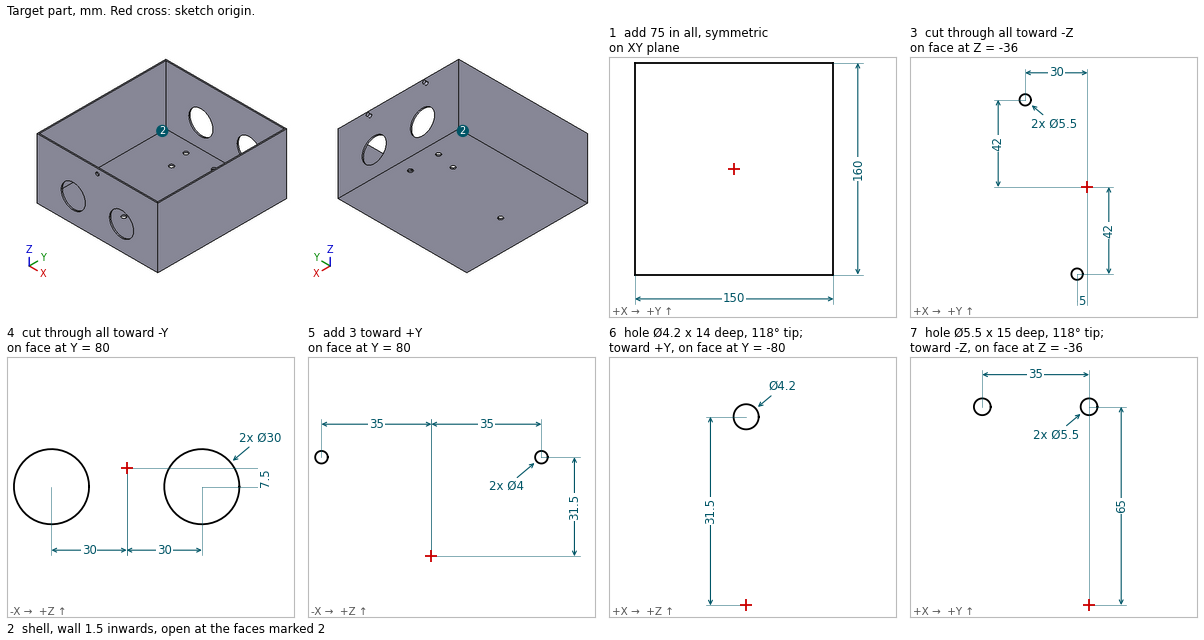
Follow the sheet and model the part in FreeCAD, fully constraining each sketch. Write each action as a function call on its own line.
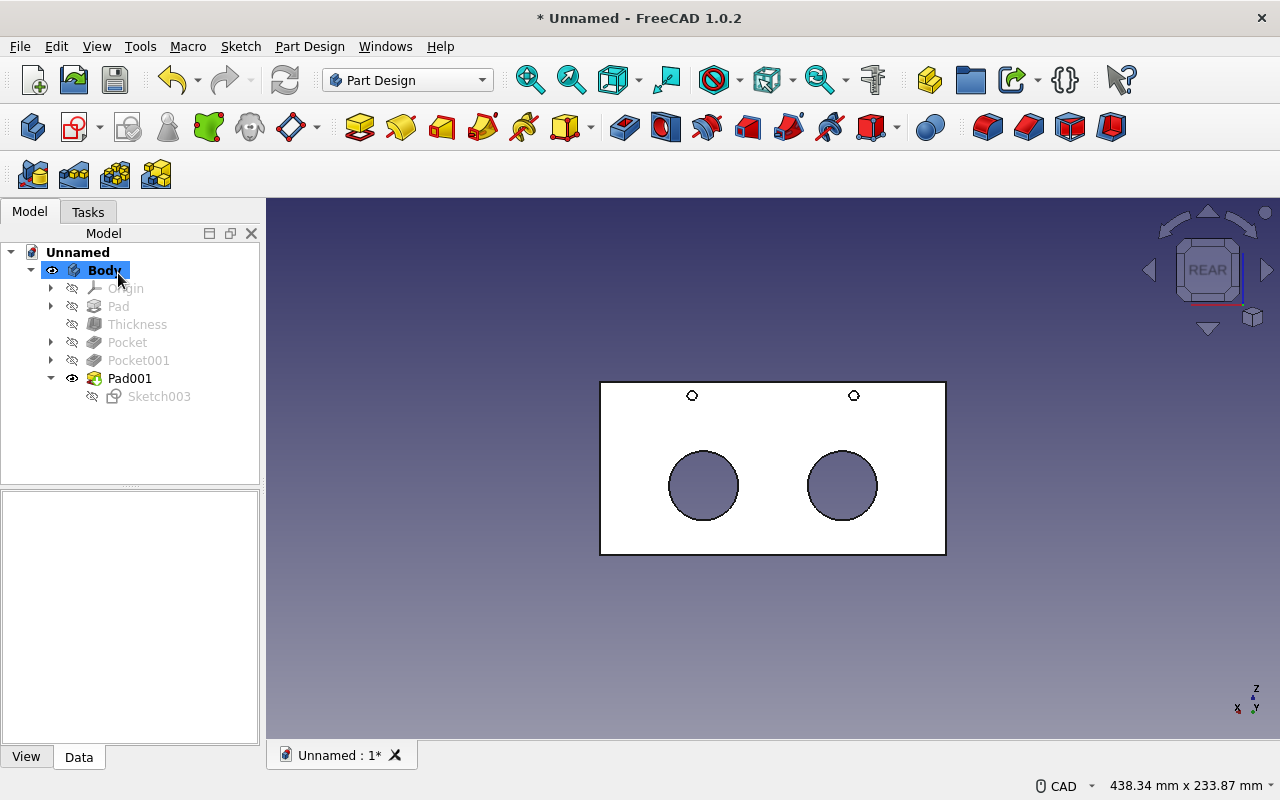
key(0)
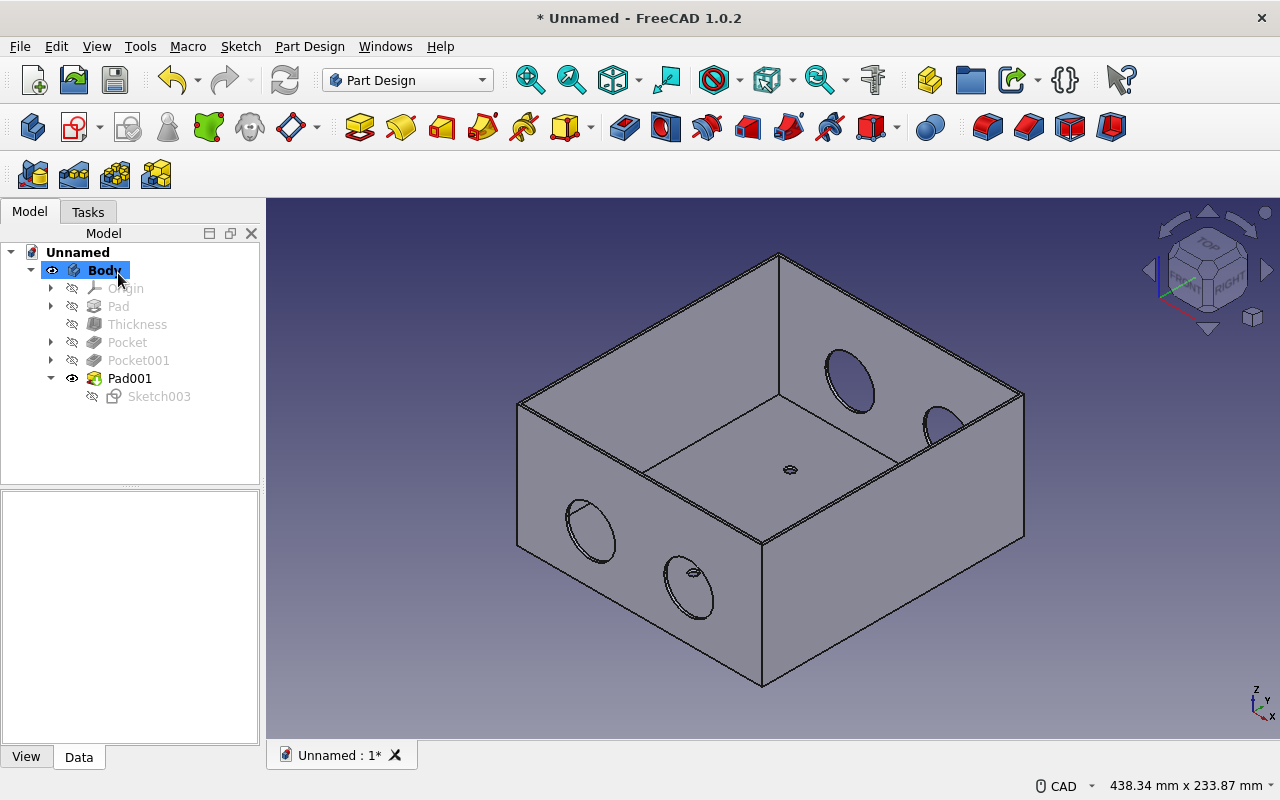
click(640, 524)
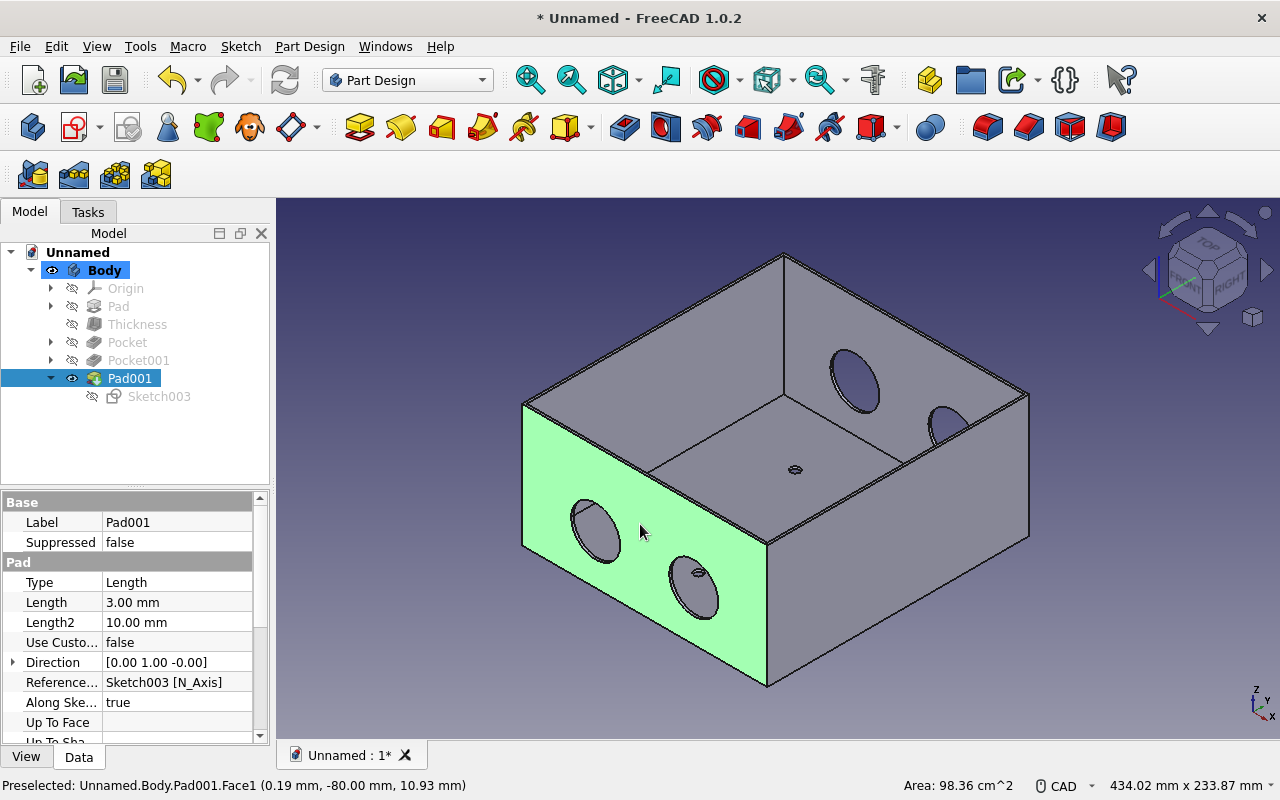
click(74, 128)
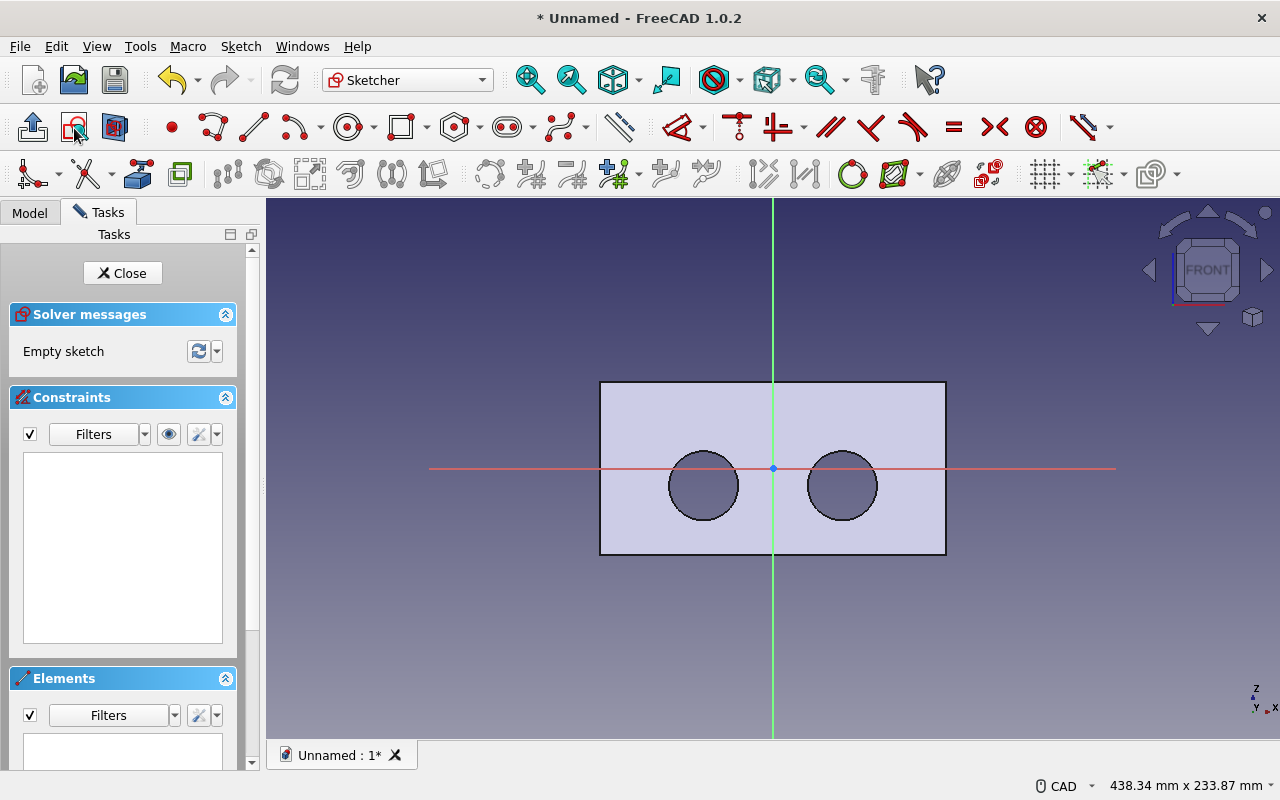
scroll(777, 392, up, 15)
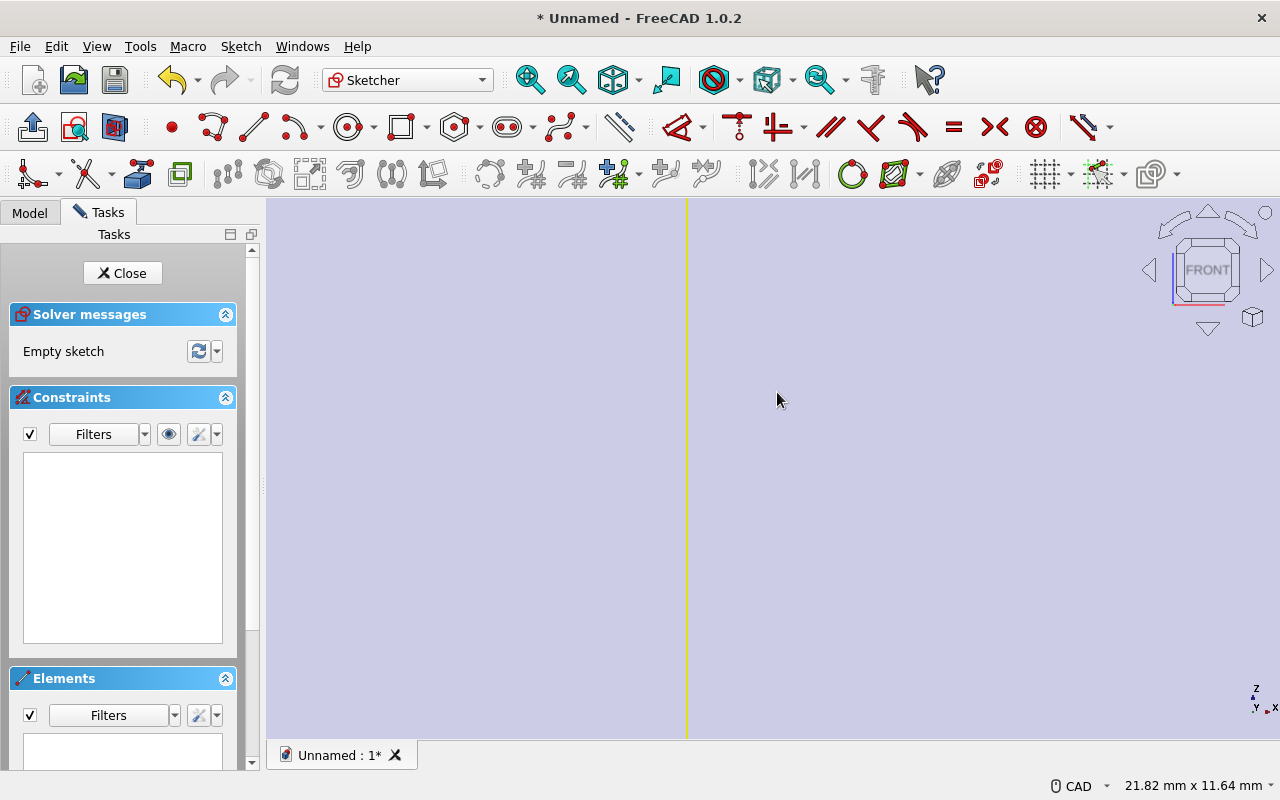
scroll(666, 445, up, 3)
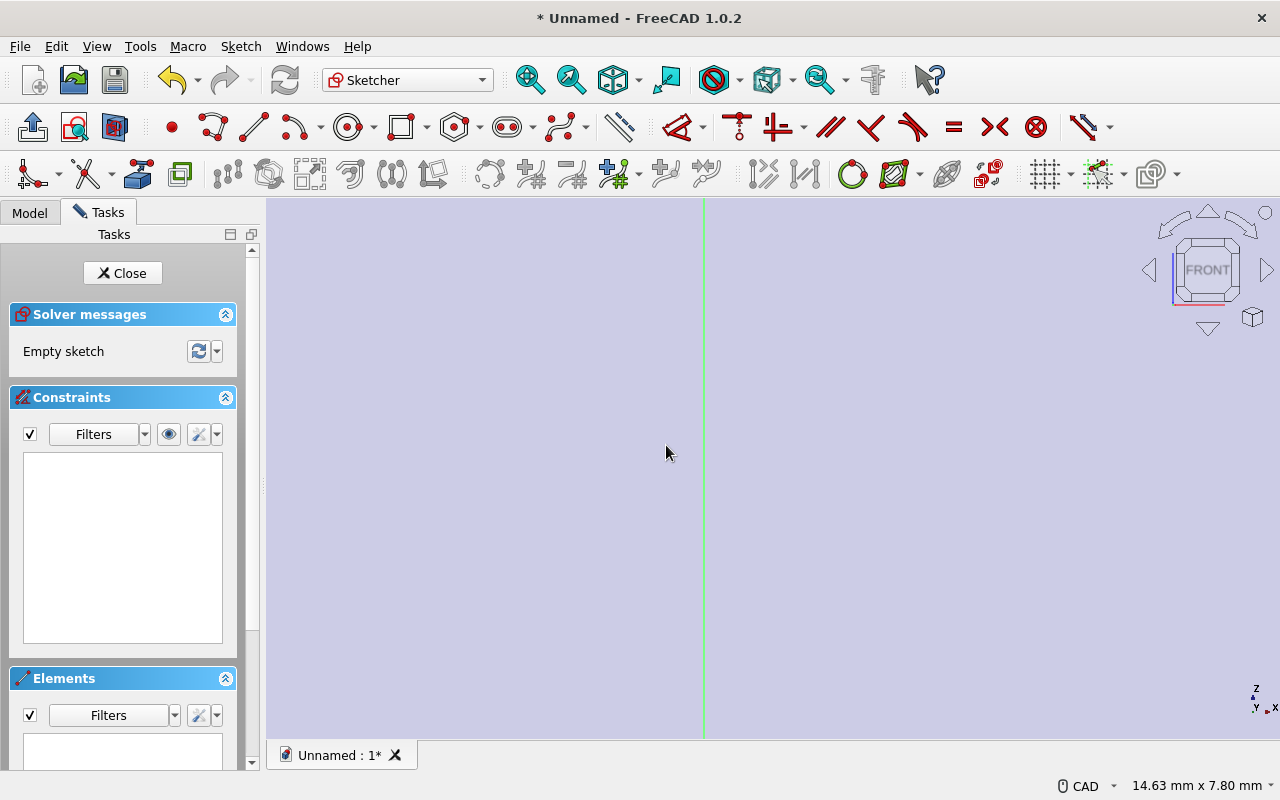
key(g)
key(c)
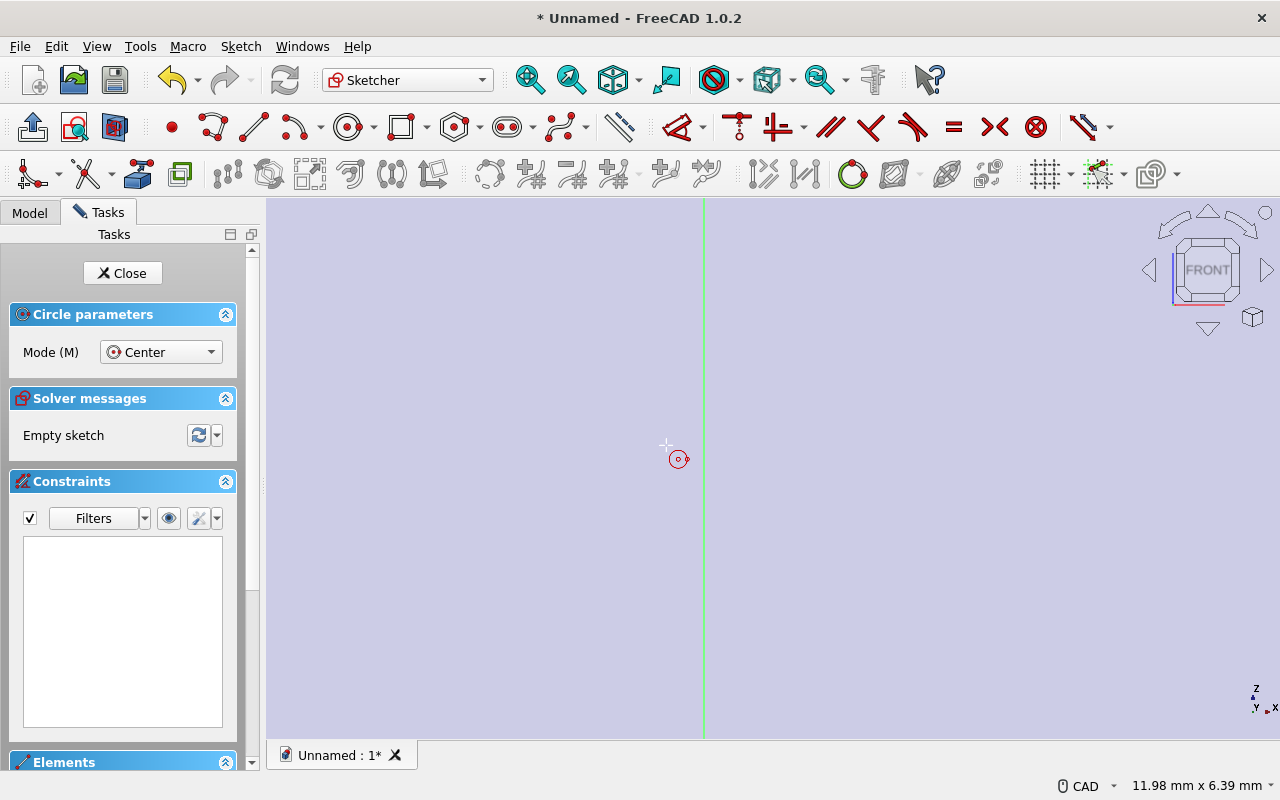
click(704, 468)
move(830, 343)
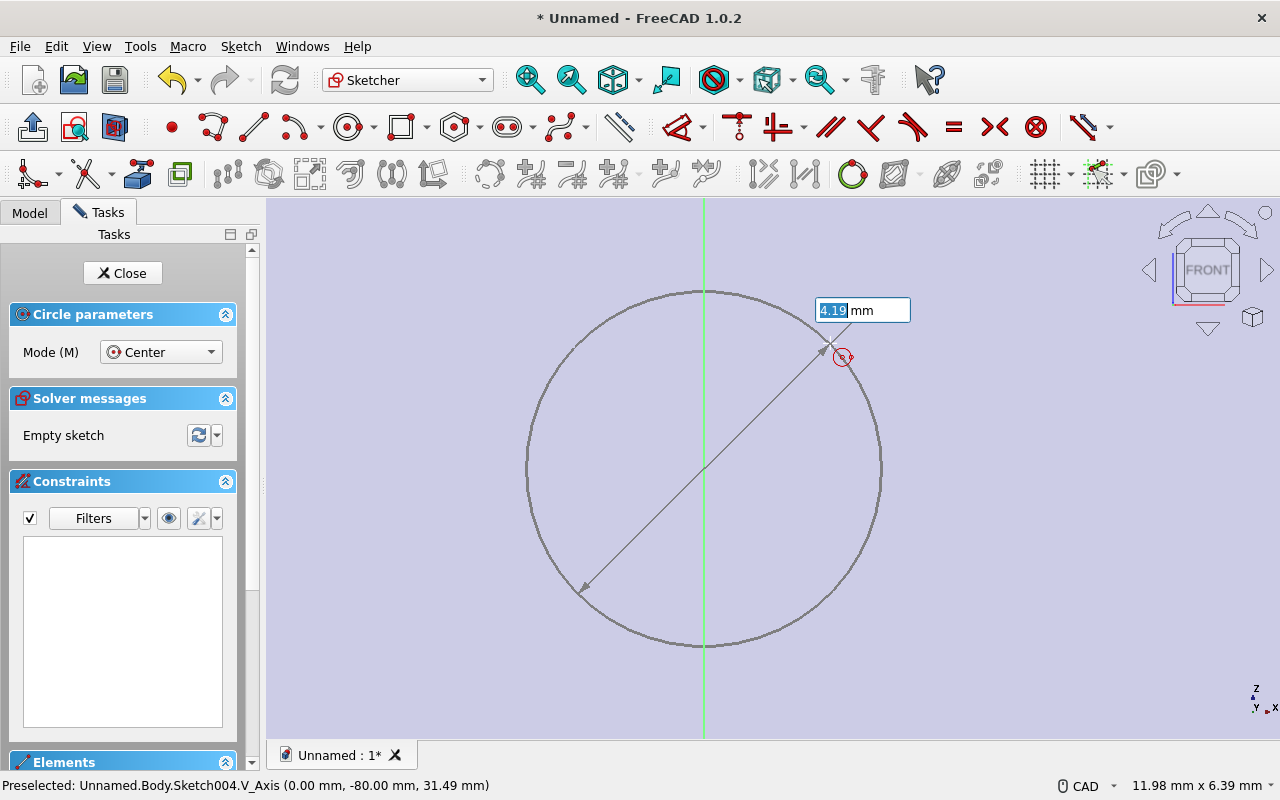
text(4.2)
key(Return)
key(Escape)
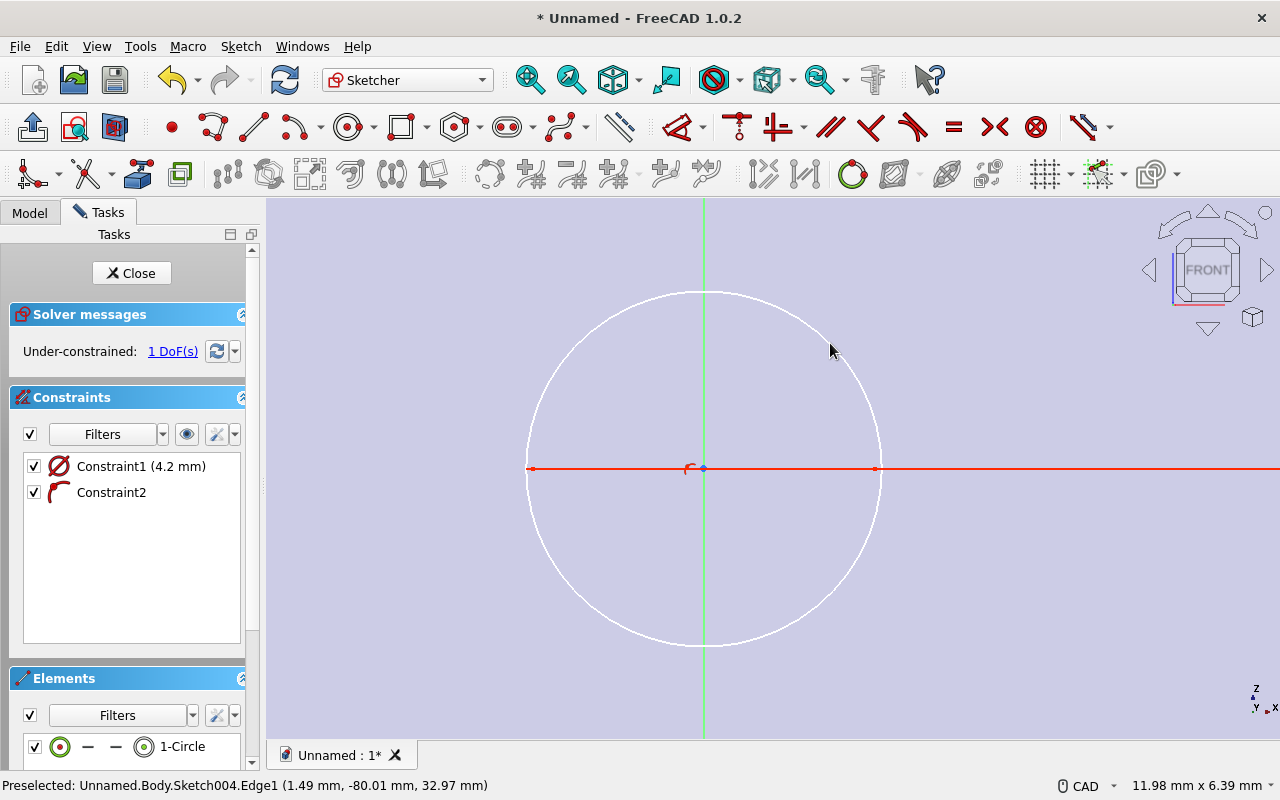
click(676, 128)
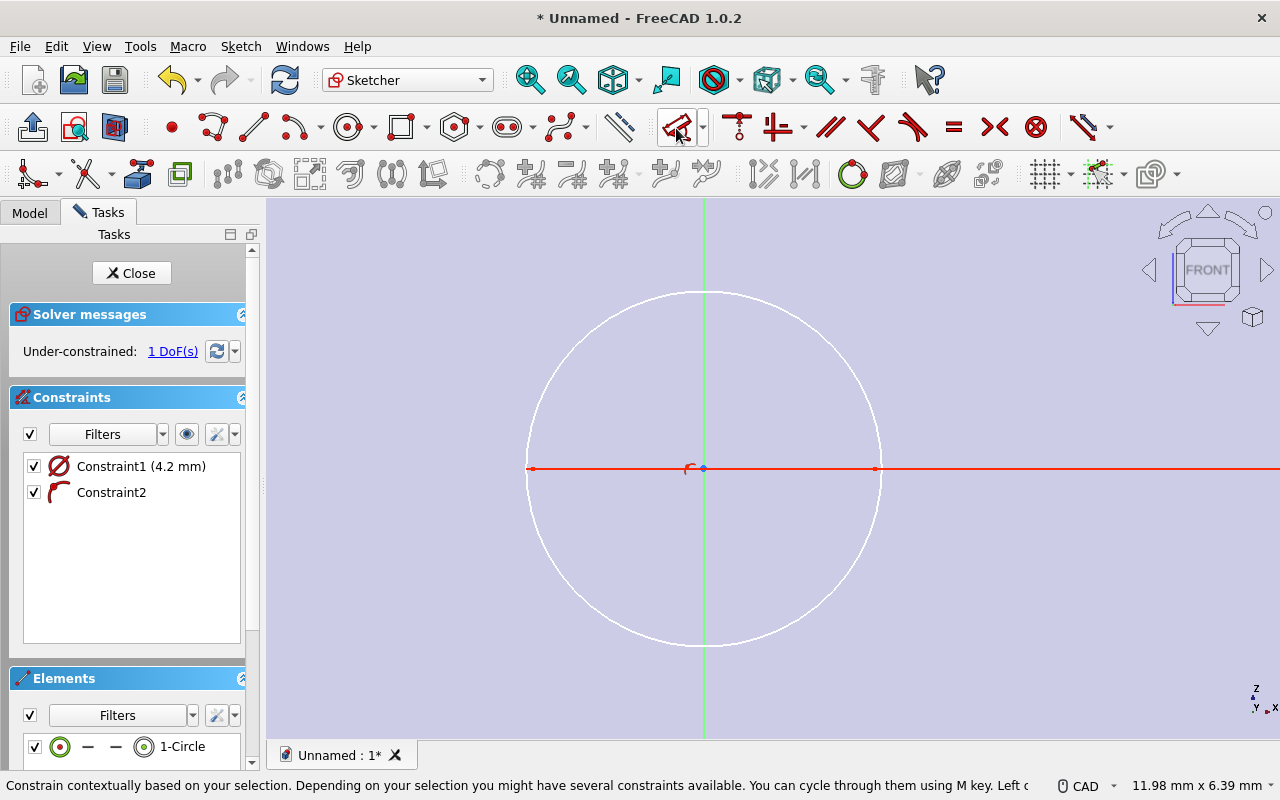
click(704, 469)
click(738, 590)